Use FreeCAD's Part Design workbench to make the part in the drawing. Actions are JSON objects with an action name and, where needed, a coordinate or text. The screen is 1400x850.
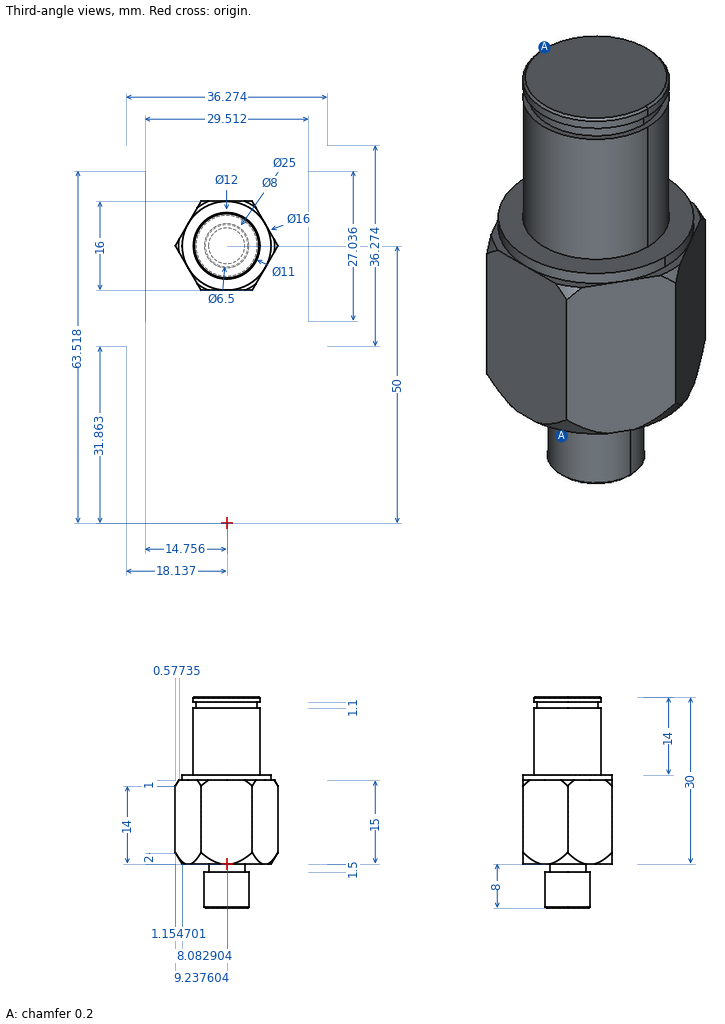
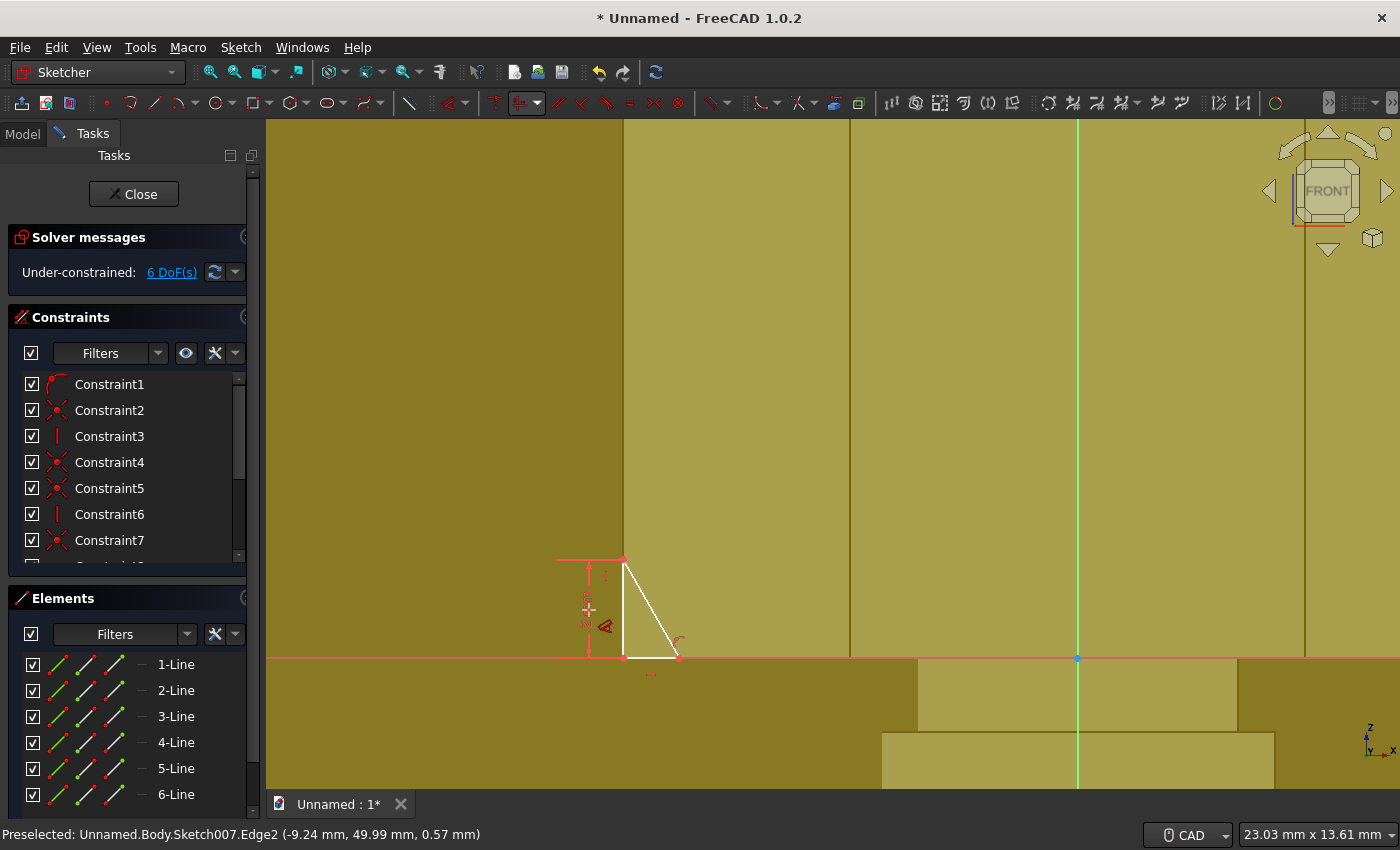
{"action": "scroll", "coordinate": [660, 655], "scroll_direction": "down", "scroll_amount": 3}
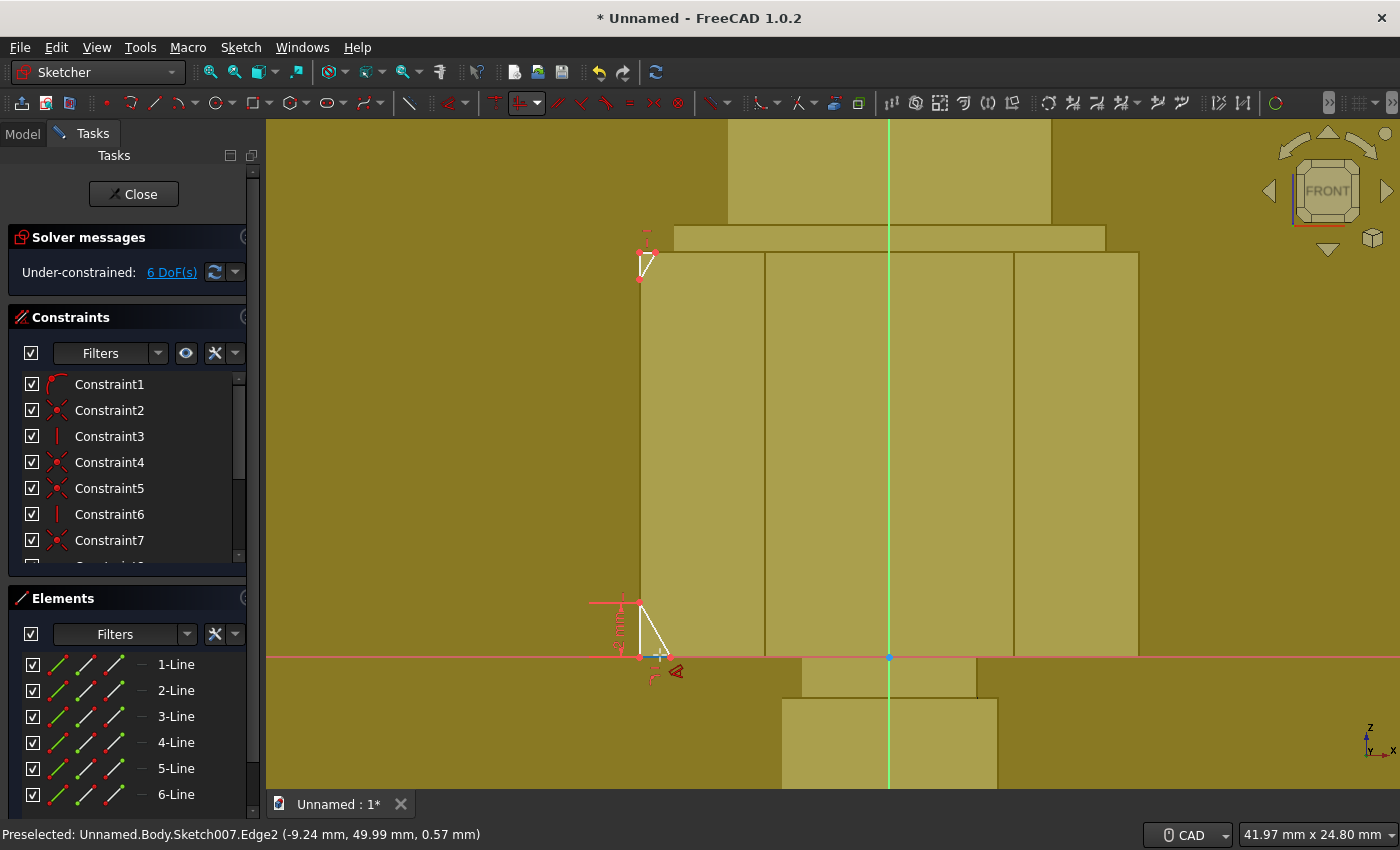
{"action": "scroll", "coordinate": [640, 261], "scroll_direction": "up", "scroll_amount": 3}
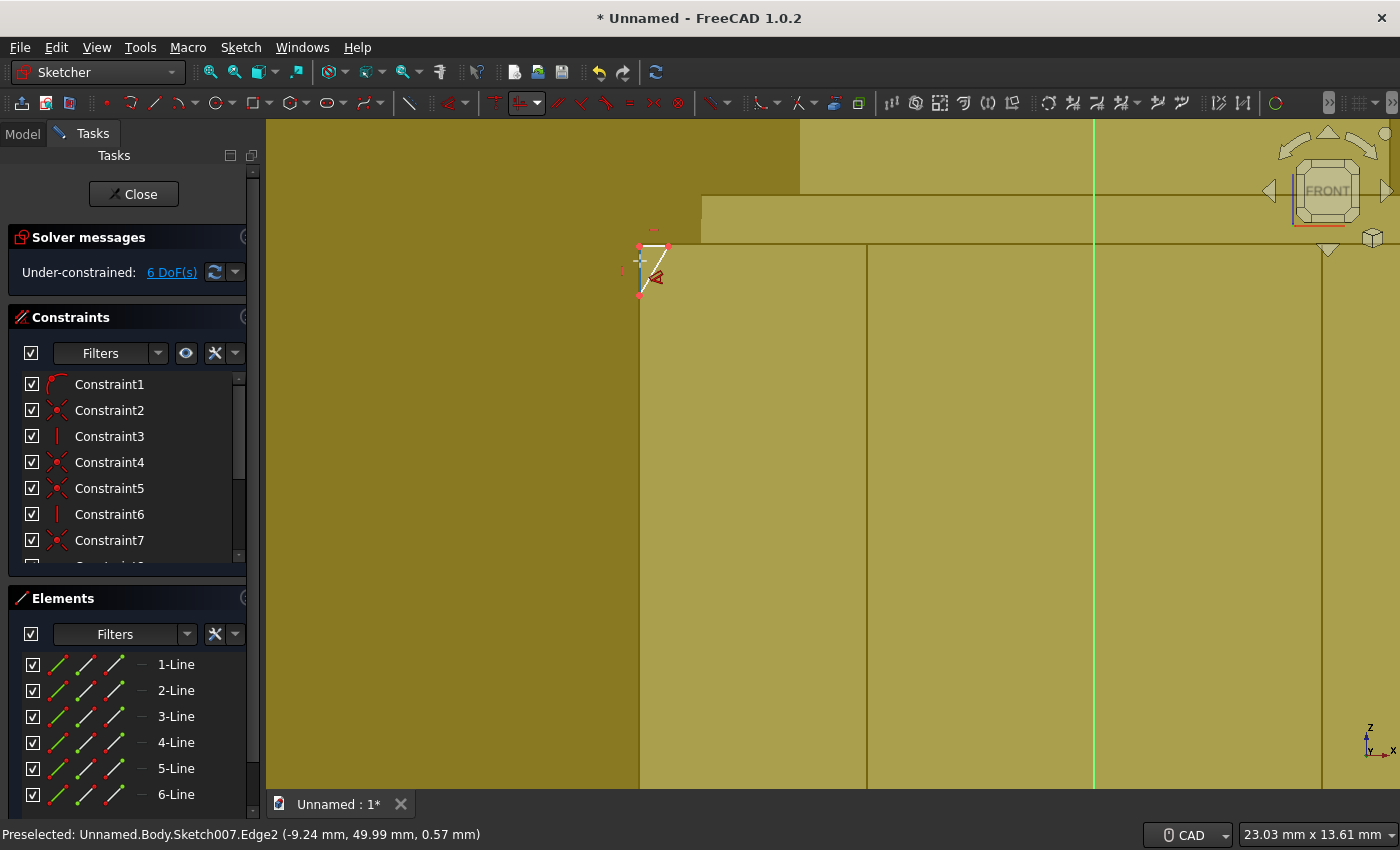
{"action": "left_click", "coordinate": [640, 261]}
{"action": "left_click", "coordinate": [606, 271]}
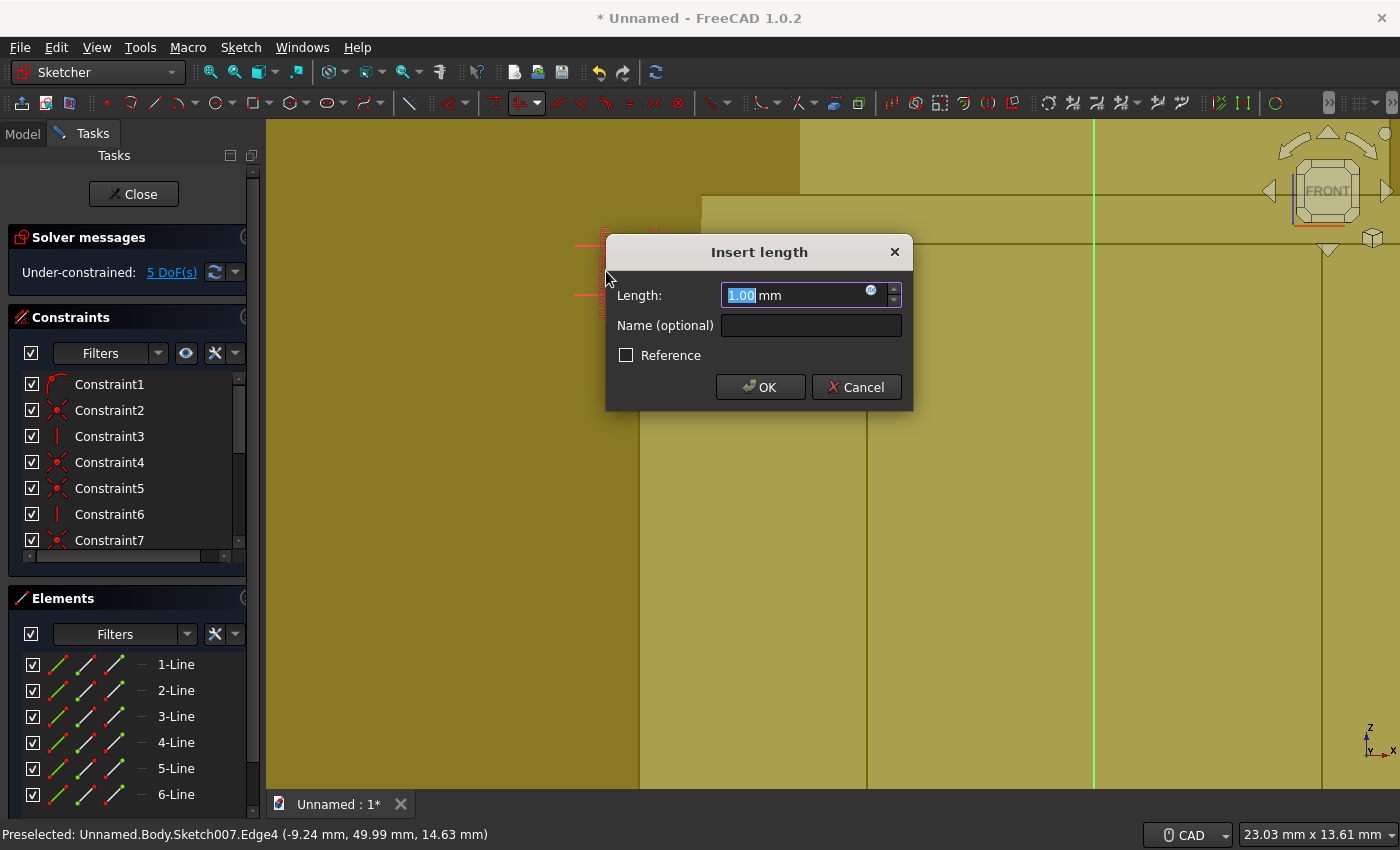
{"action": "type", "text": "1"}
{"action": "key", "text": "Return"}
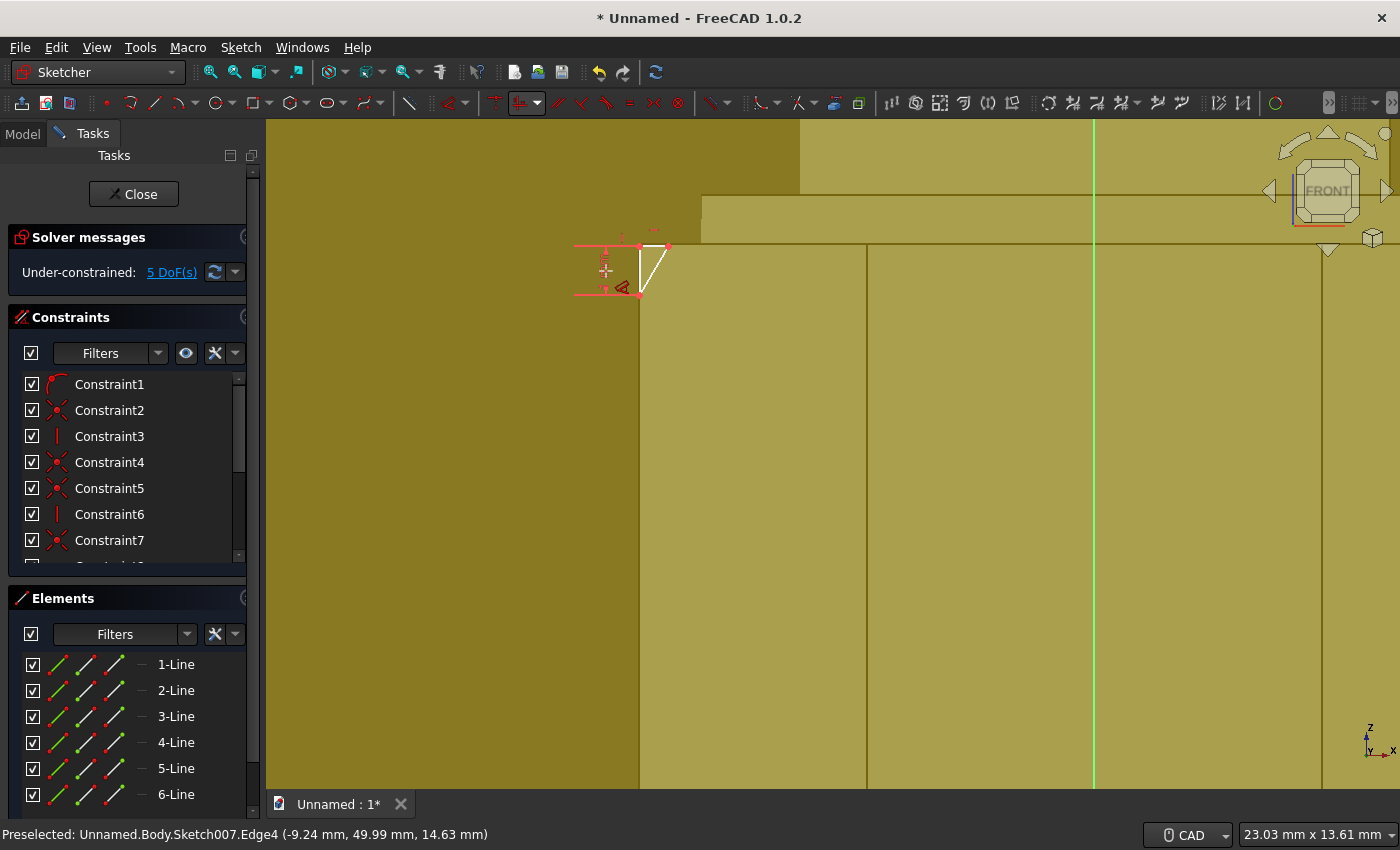
{"action": "left_click", "coordinate": [640, 295]}
{"action": "left_click", "coordinate": [1128, 528]}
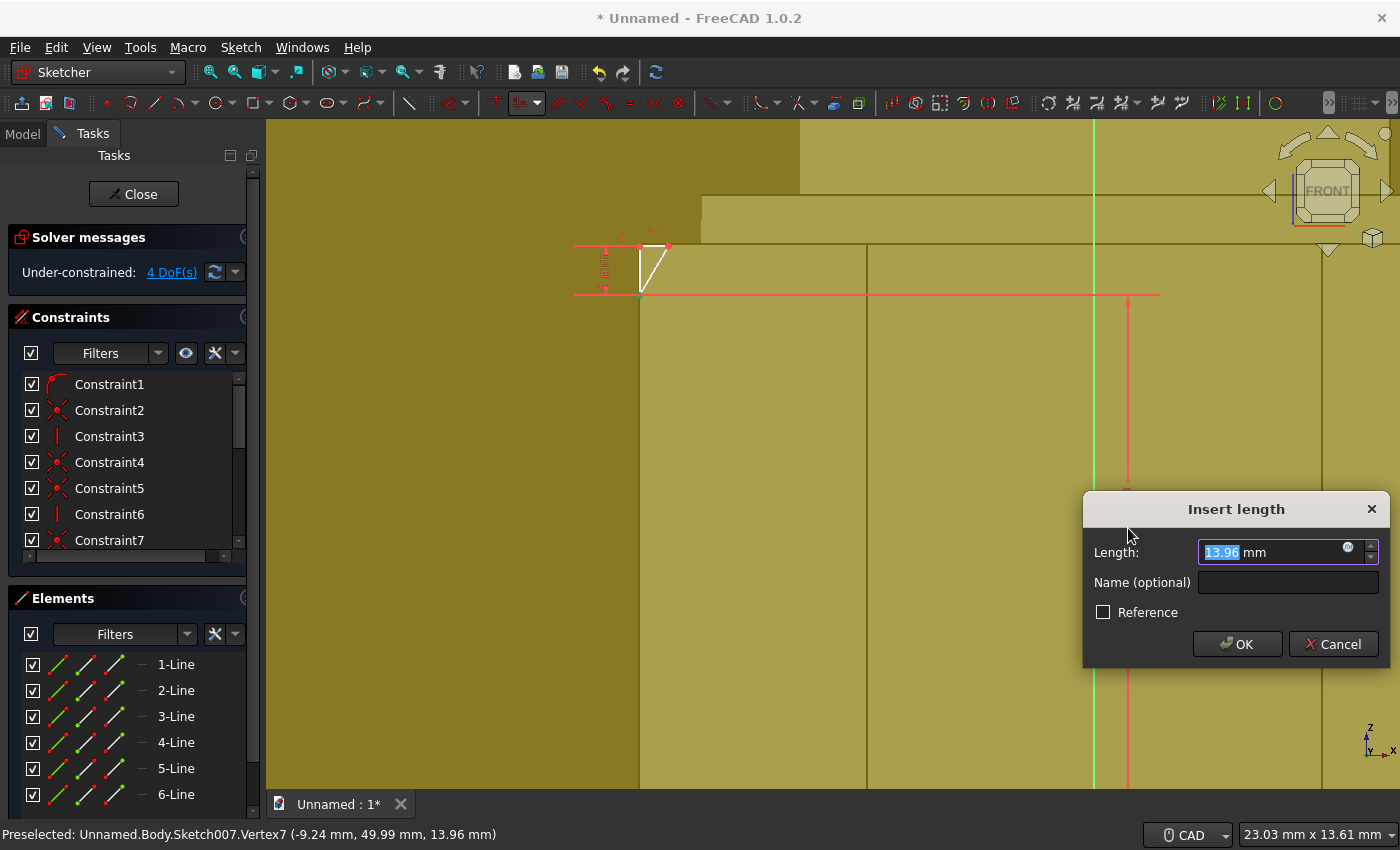
{"action": "type", "text": "14"}
{"action": "key", "text": "Return"}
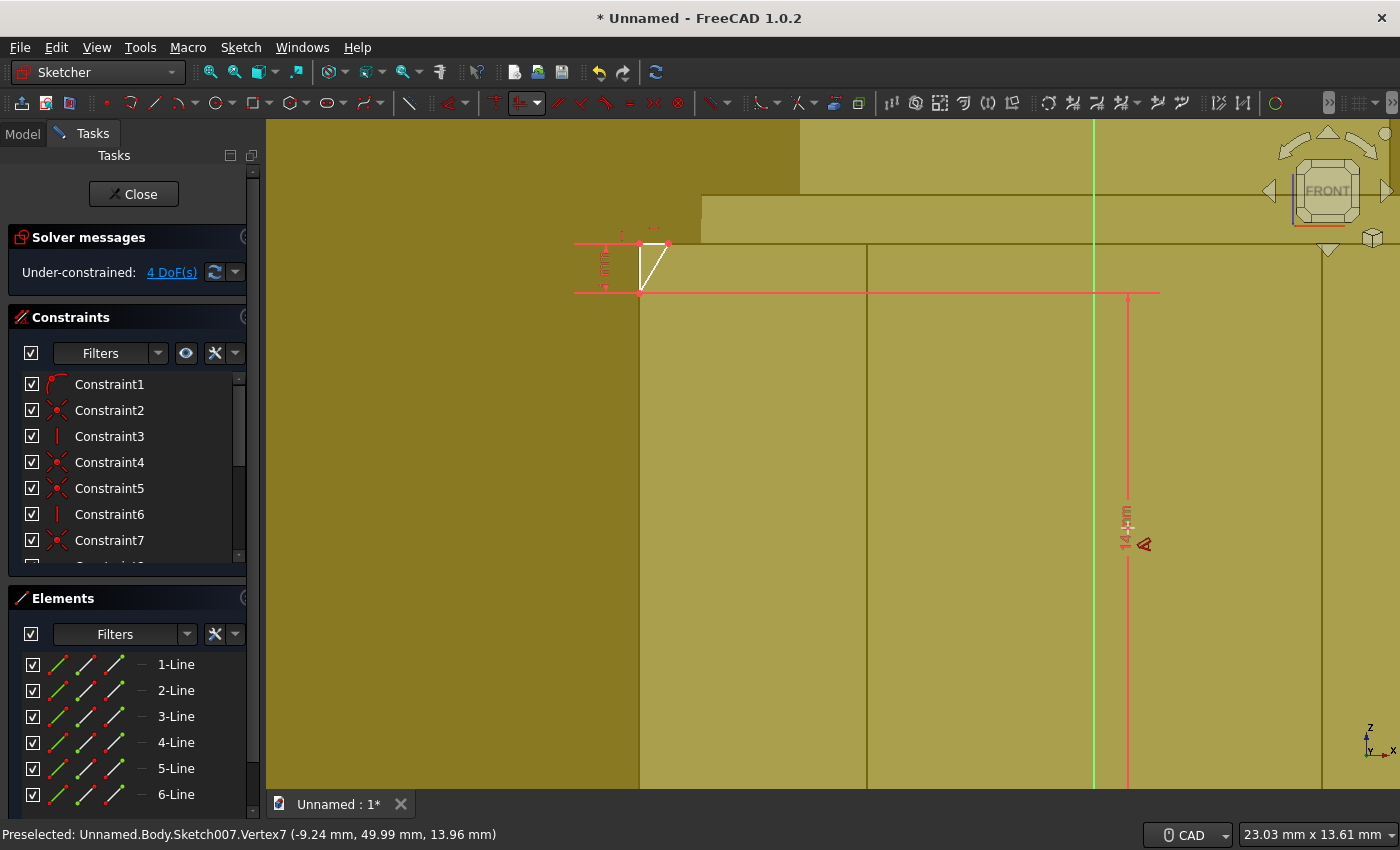
{"action": "scroll", "coordinate": [651, 244], "scroll_direction": "up", "scroll_amount": 2}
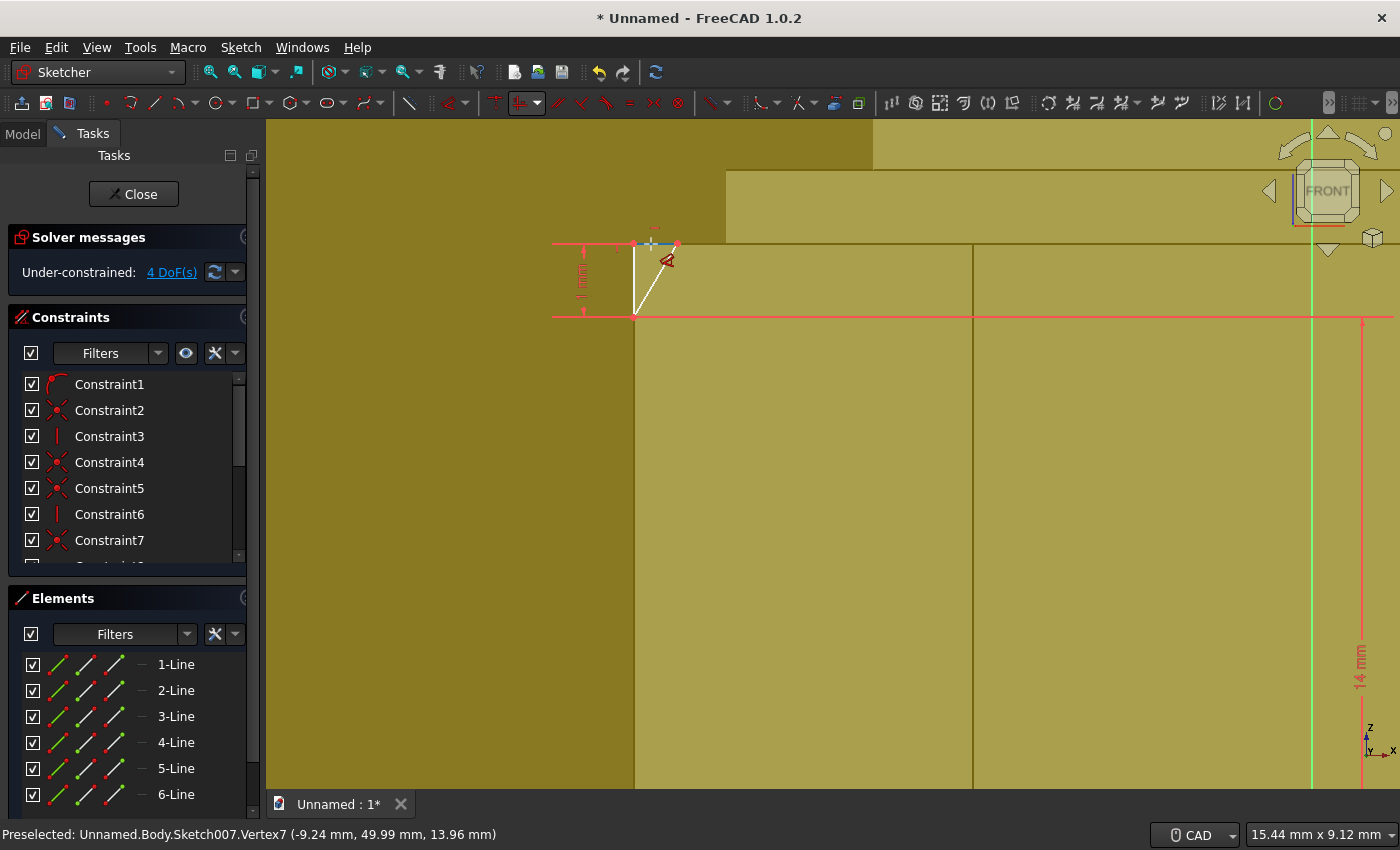
{"action": "left_click", "coordinate": [651, 244]}
{"action": "left_click", "coordinate": [656, 210]}